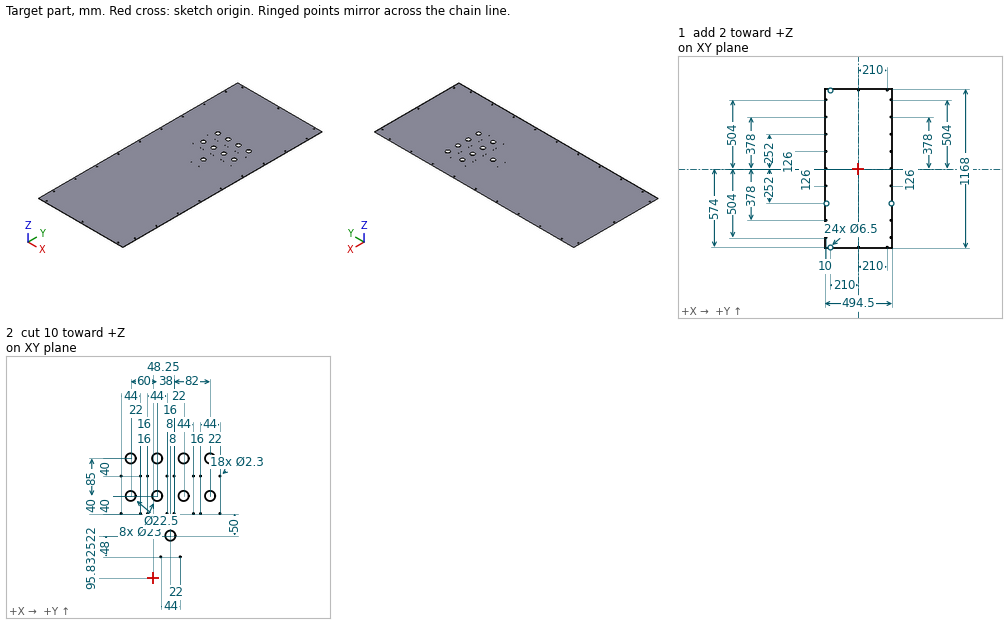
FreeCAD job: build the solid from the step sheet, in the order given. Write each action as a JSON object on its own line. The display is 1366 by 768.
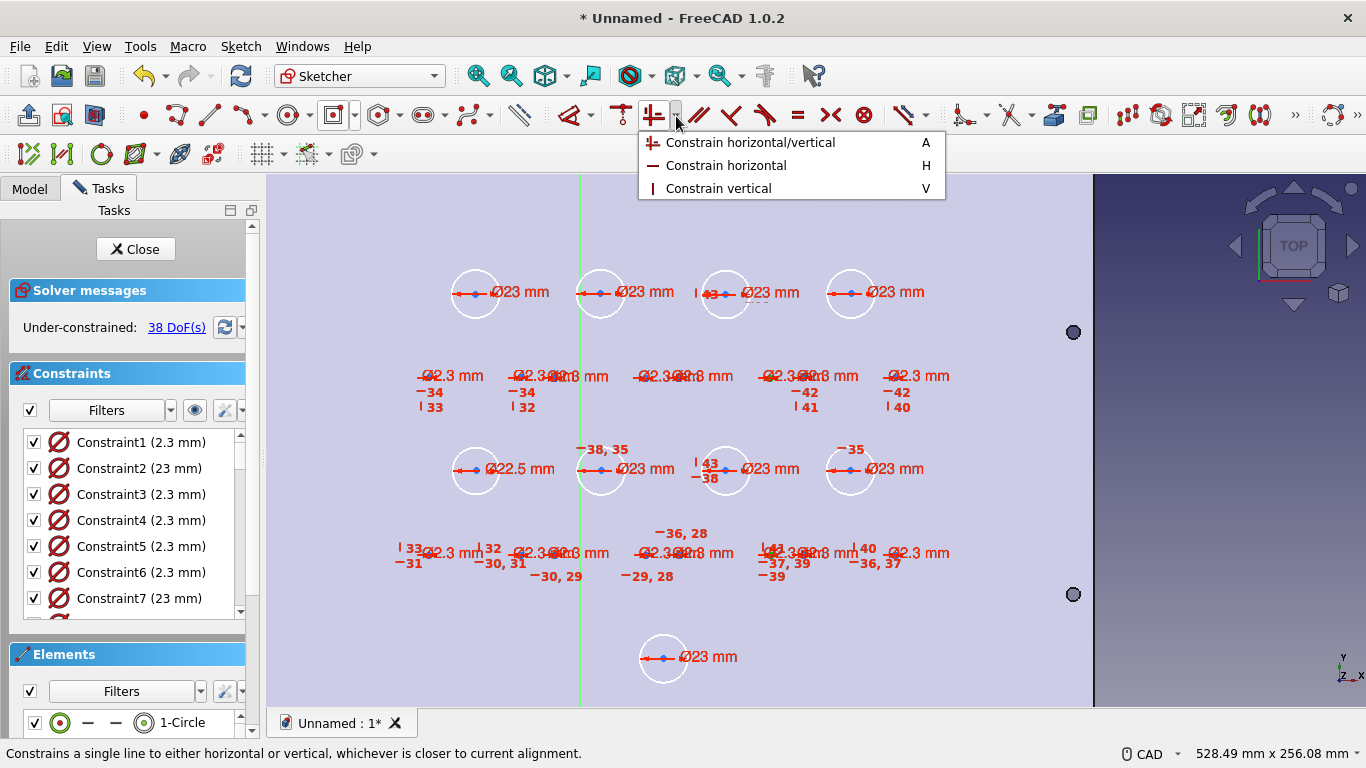
{"action": "left_click", "coordinate": [792, 188]}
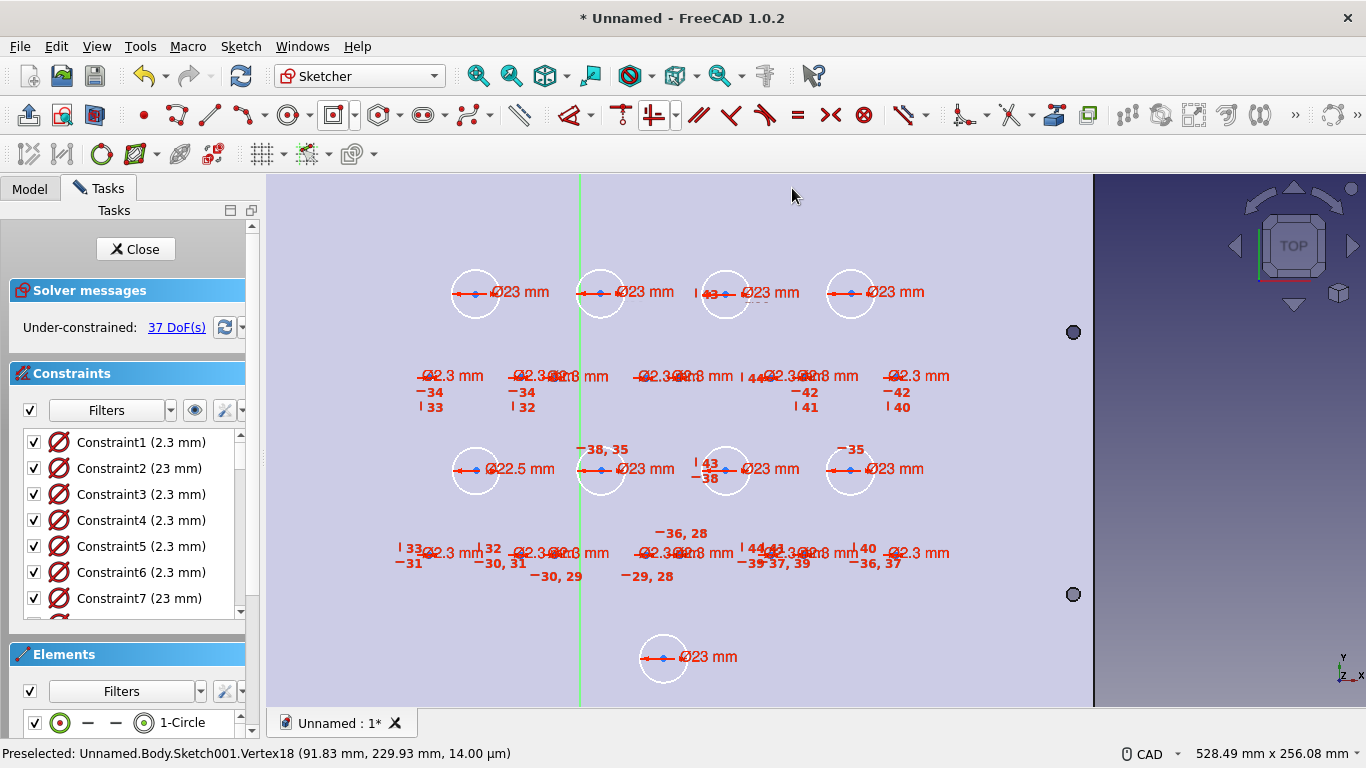
{"action": "left_click", "coordinate": [805, 378]}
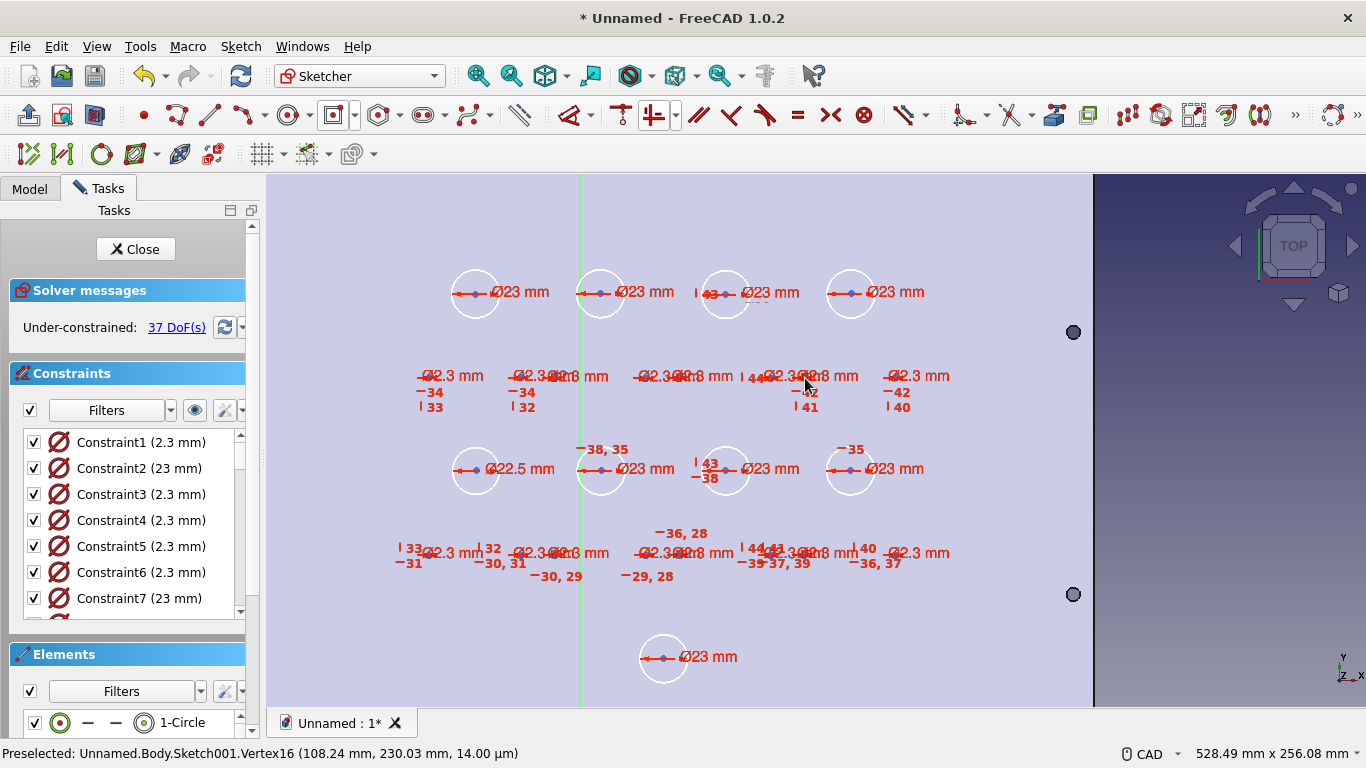
{"action": "left_click", "coordinate": [771, 378]}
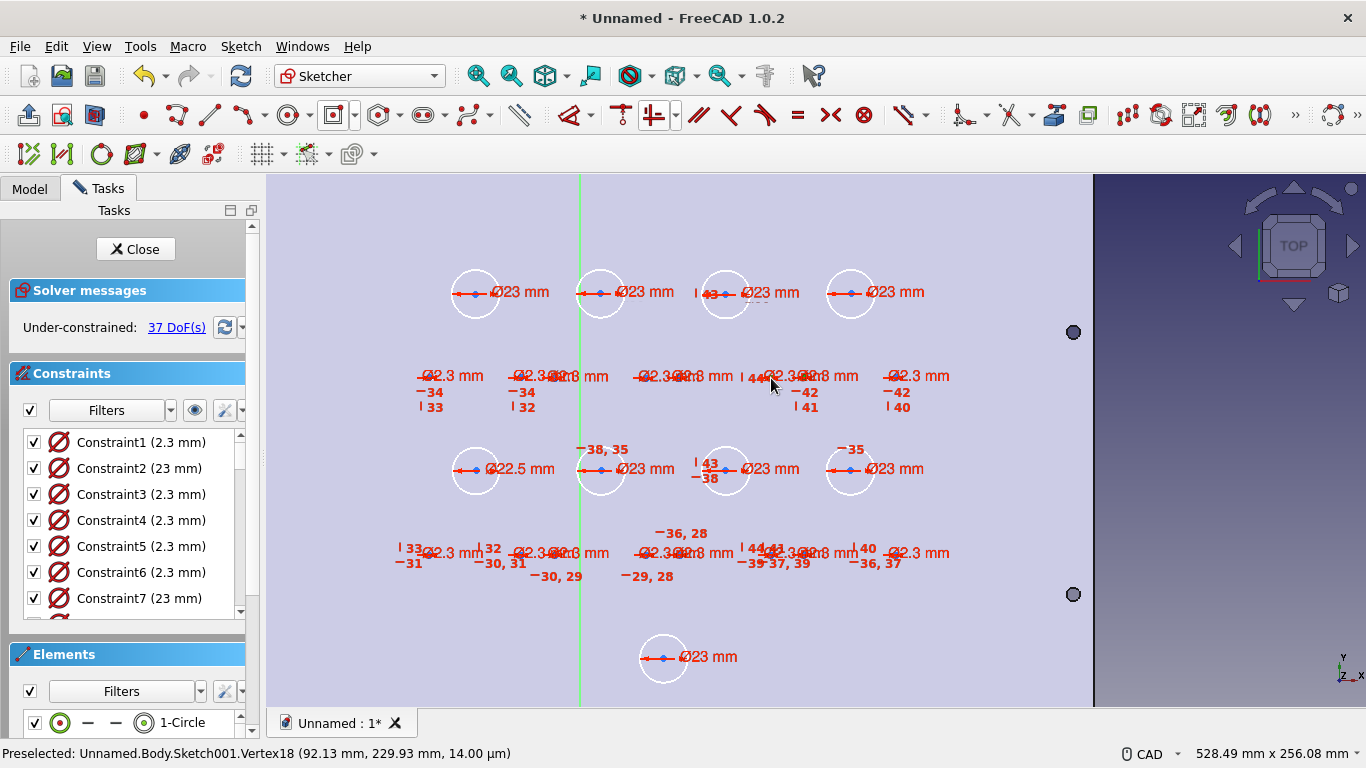
{"action": "left_click", "coordinate": [676, 116]}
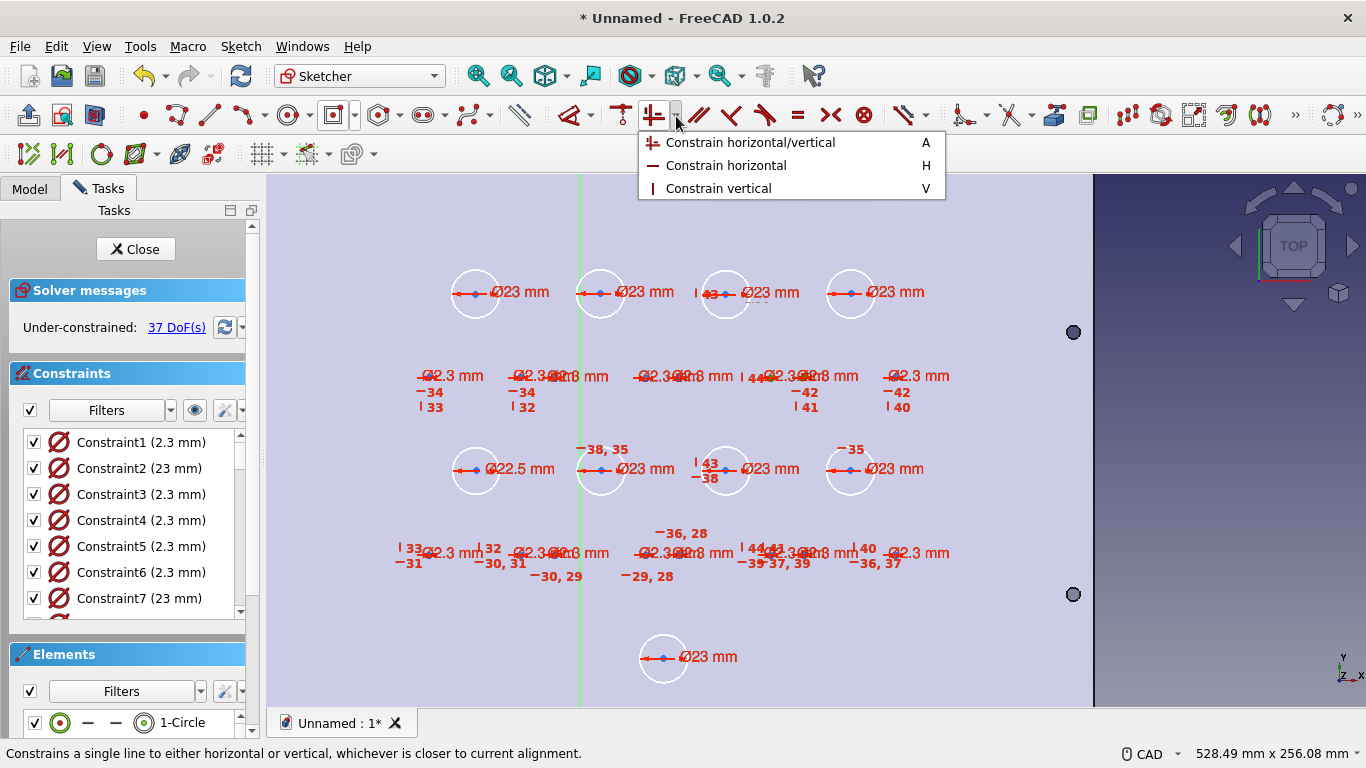
{"action": "left_click", "coordinate": [792, 166]}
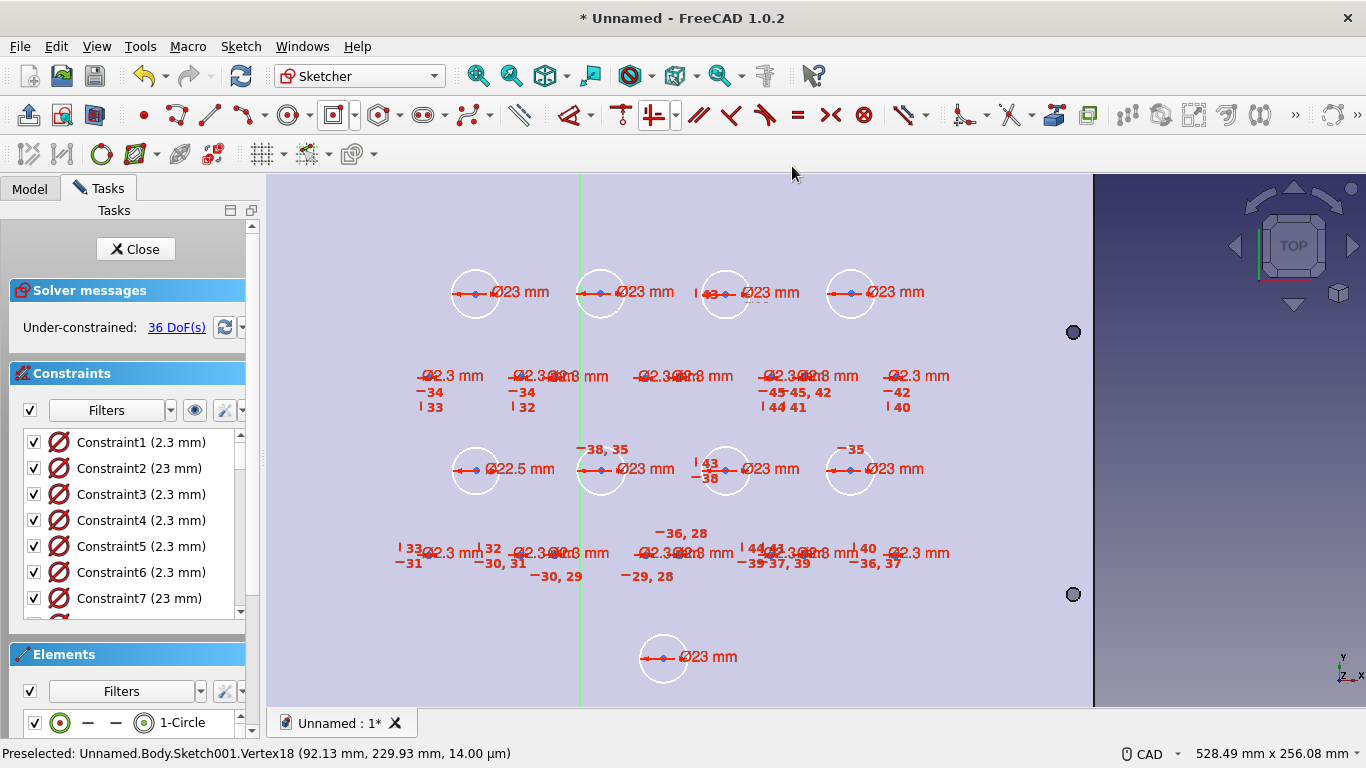
{"action": "left_click", "coordinate": [771, 378]}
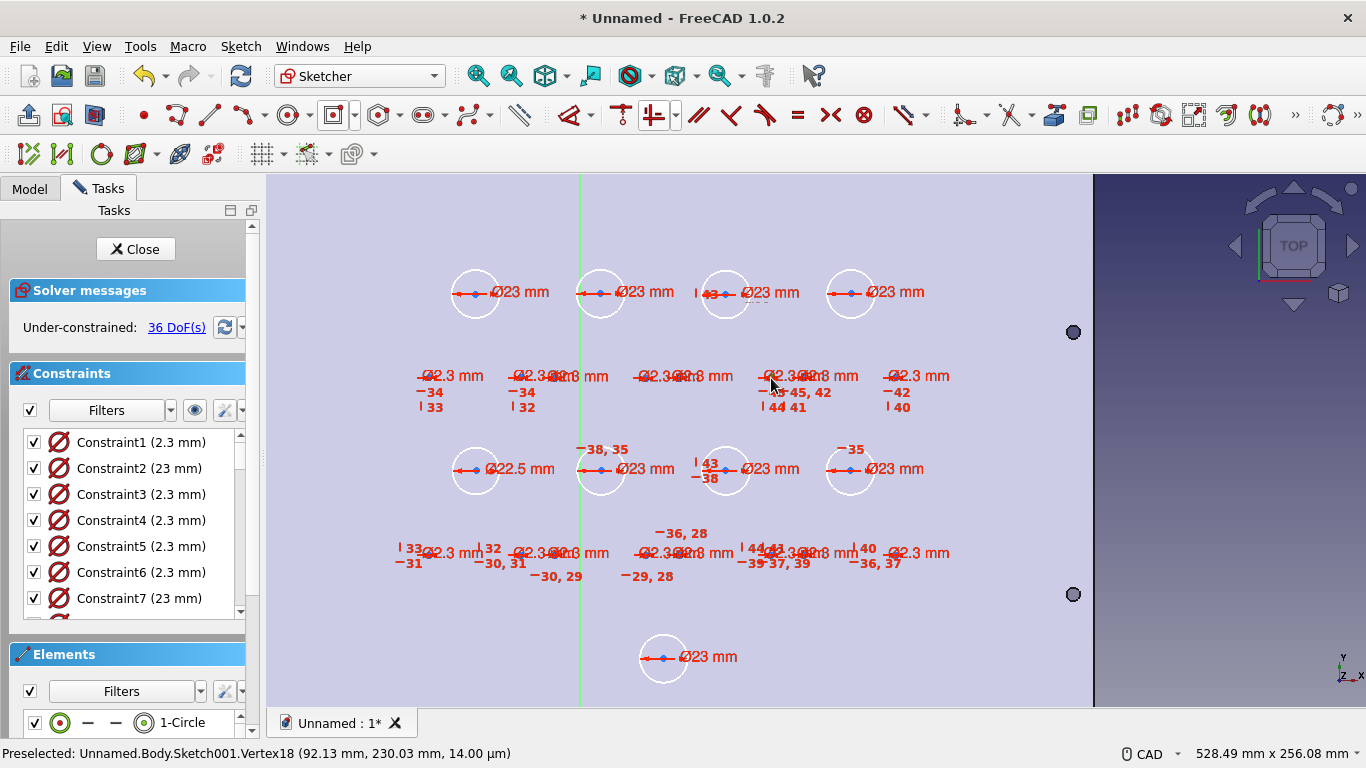
{"action": "left_click", "coordinate": [680, 378]}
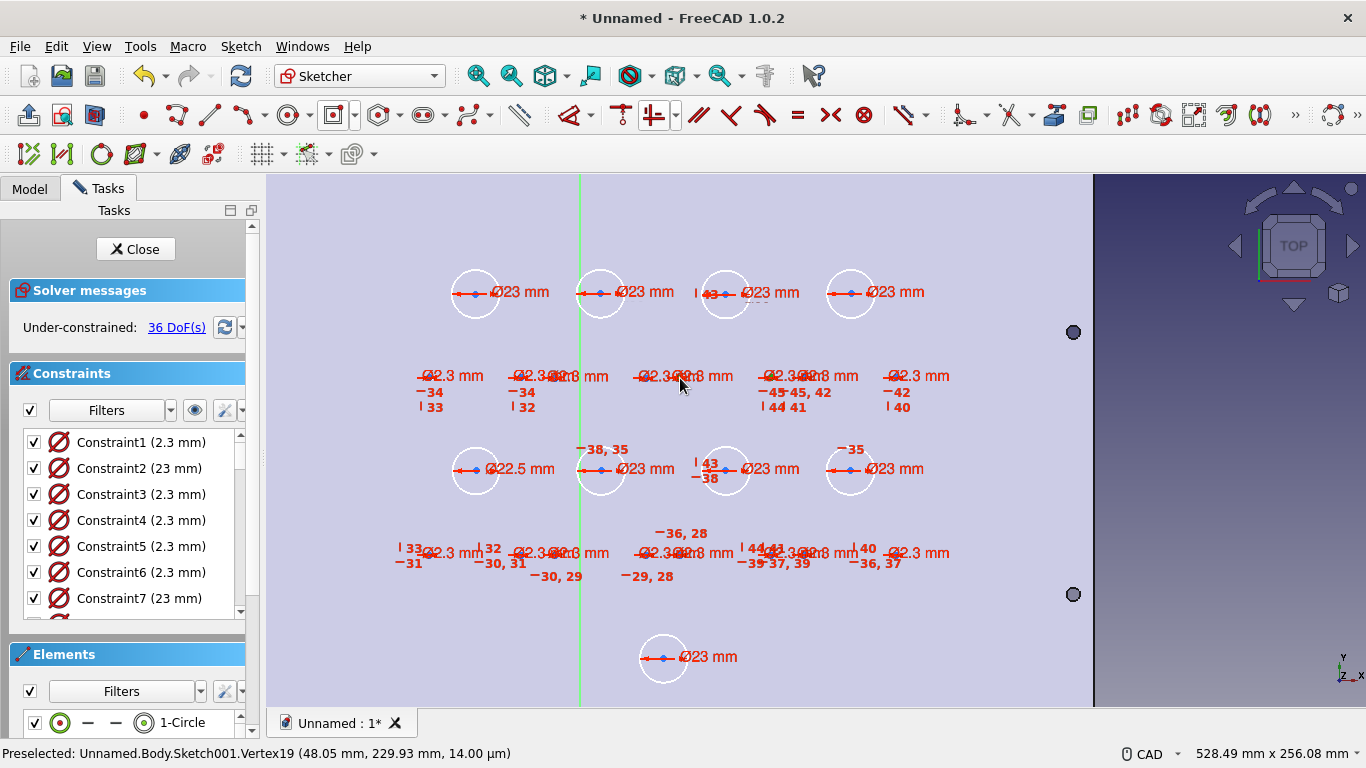
{"action": "key", "text": "h"}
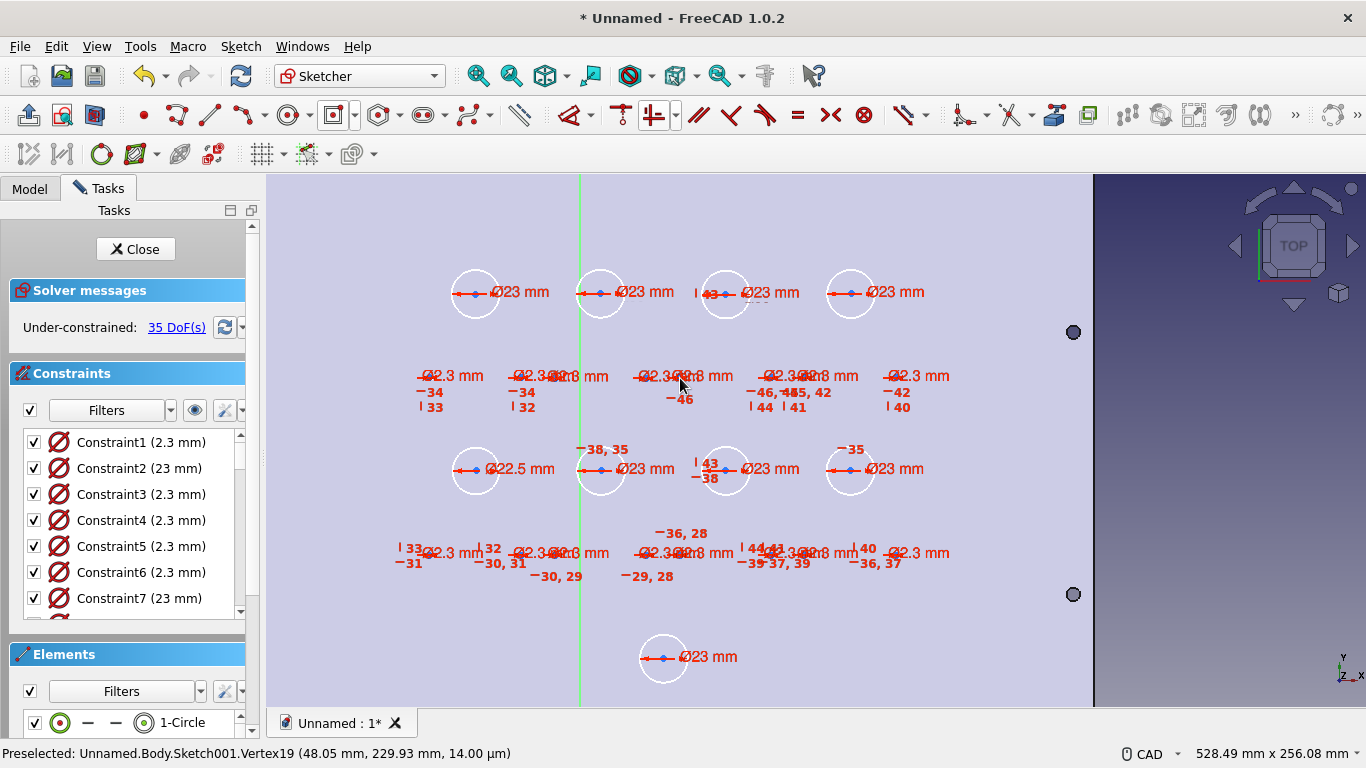
{"action": "left_click", "coordinate": [521, 378]}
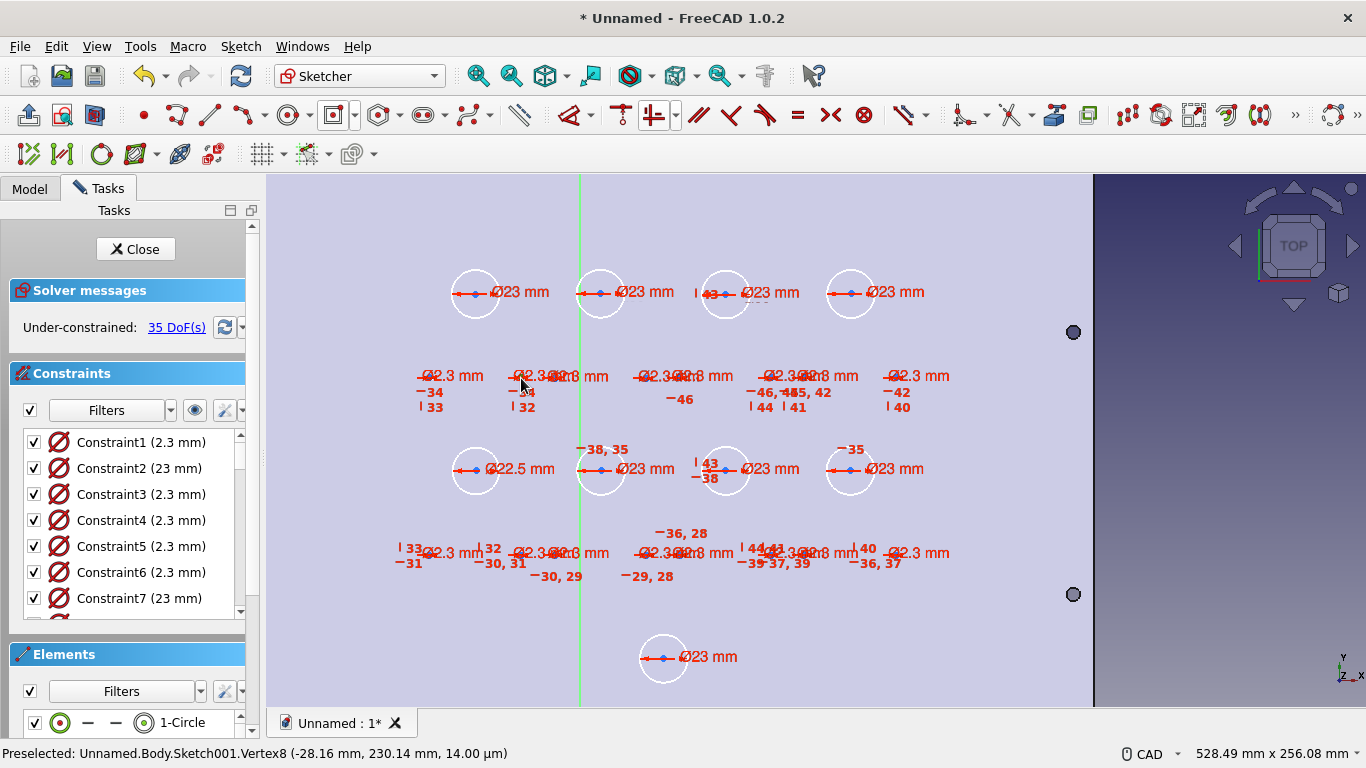
{"action": "left_click", "coordinate": [680, 378]}